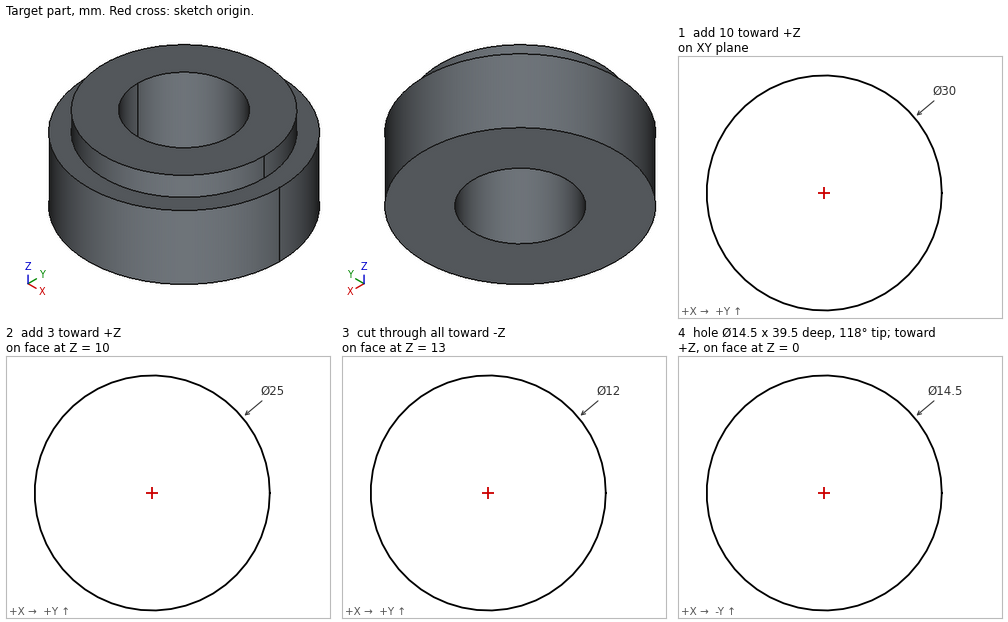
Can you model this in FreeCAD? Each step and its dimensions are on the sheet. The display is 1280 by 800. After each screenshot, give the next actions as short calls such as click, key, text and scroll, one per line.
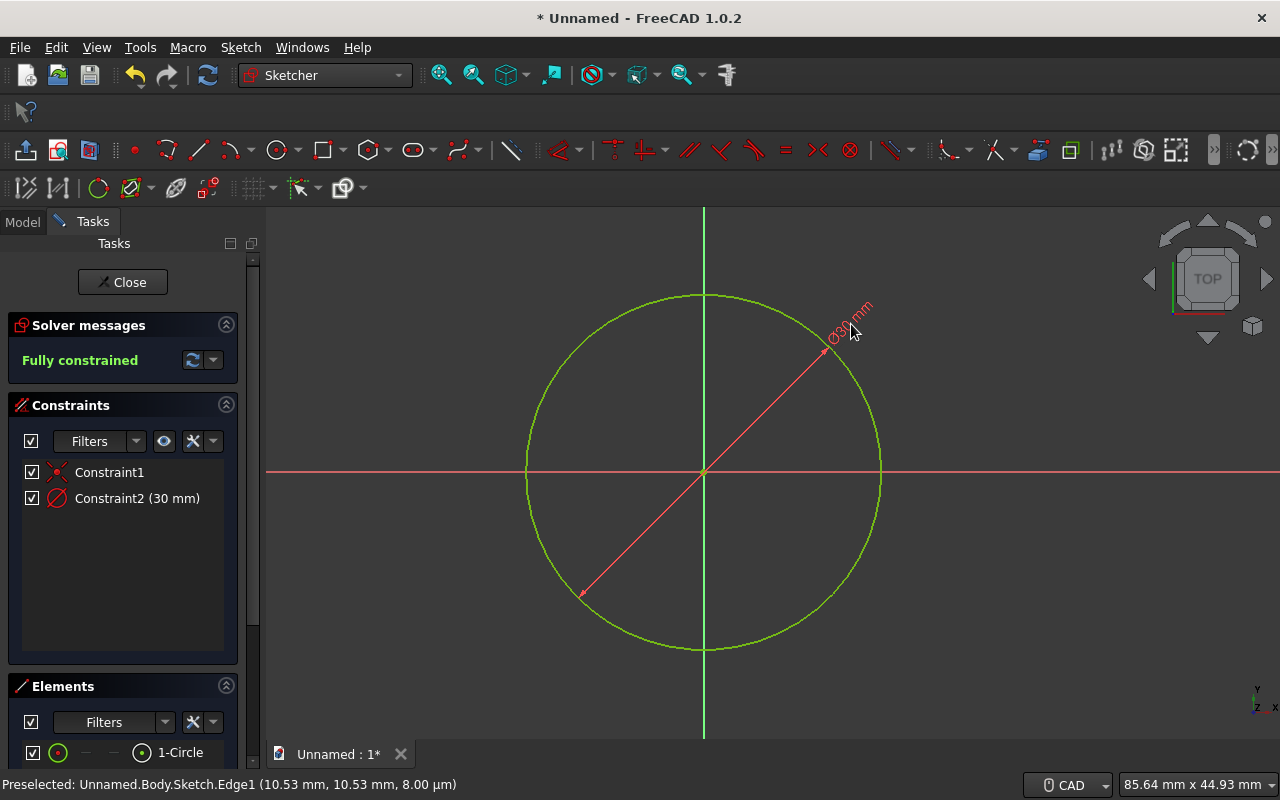
click(123, 282)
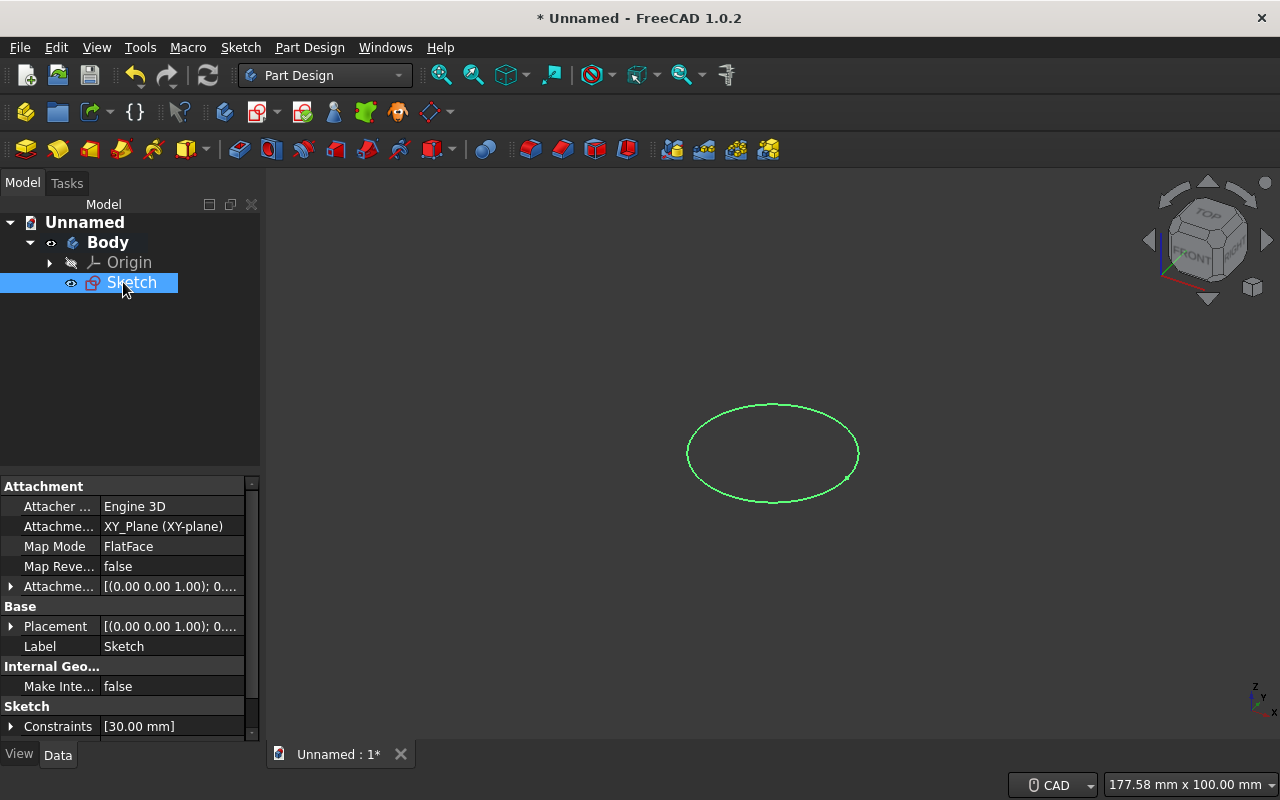
click(26, 150)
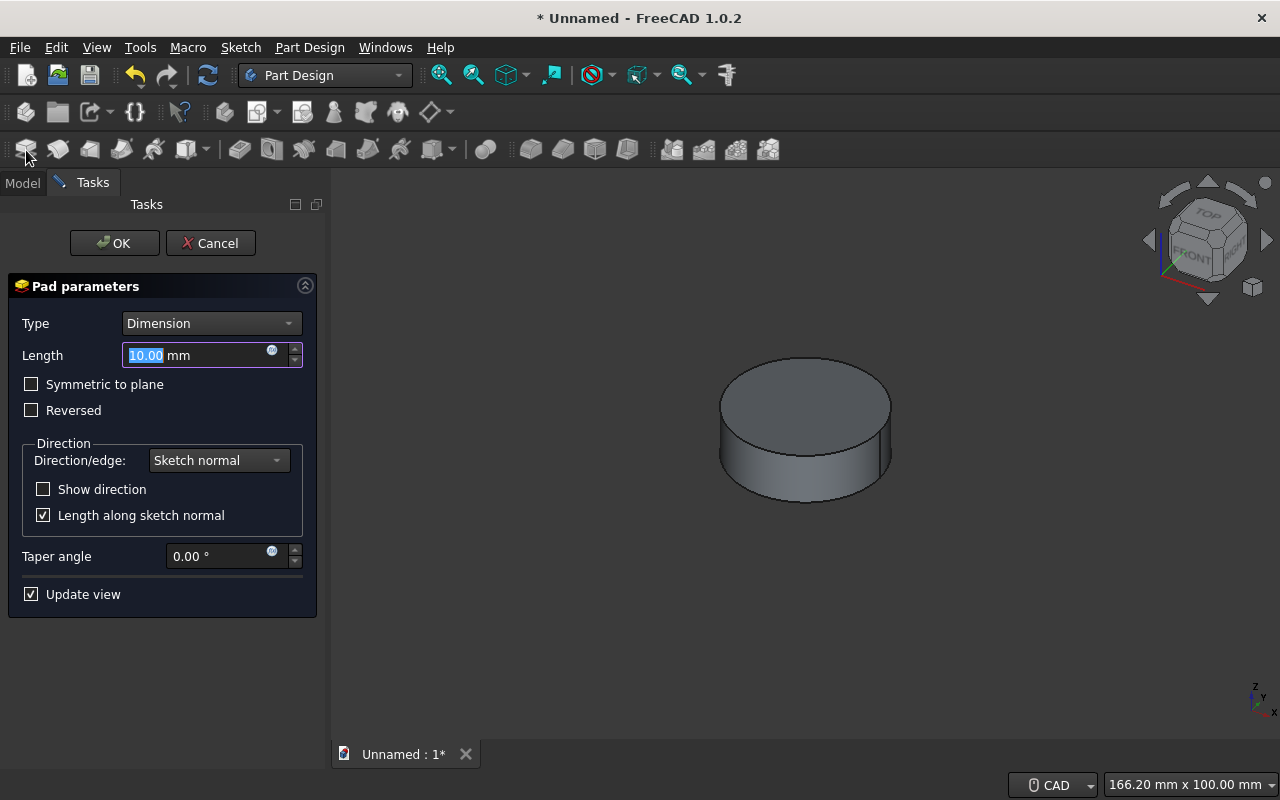
text(10)
key(Tab)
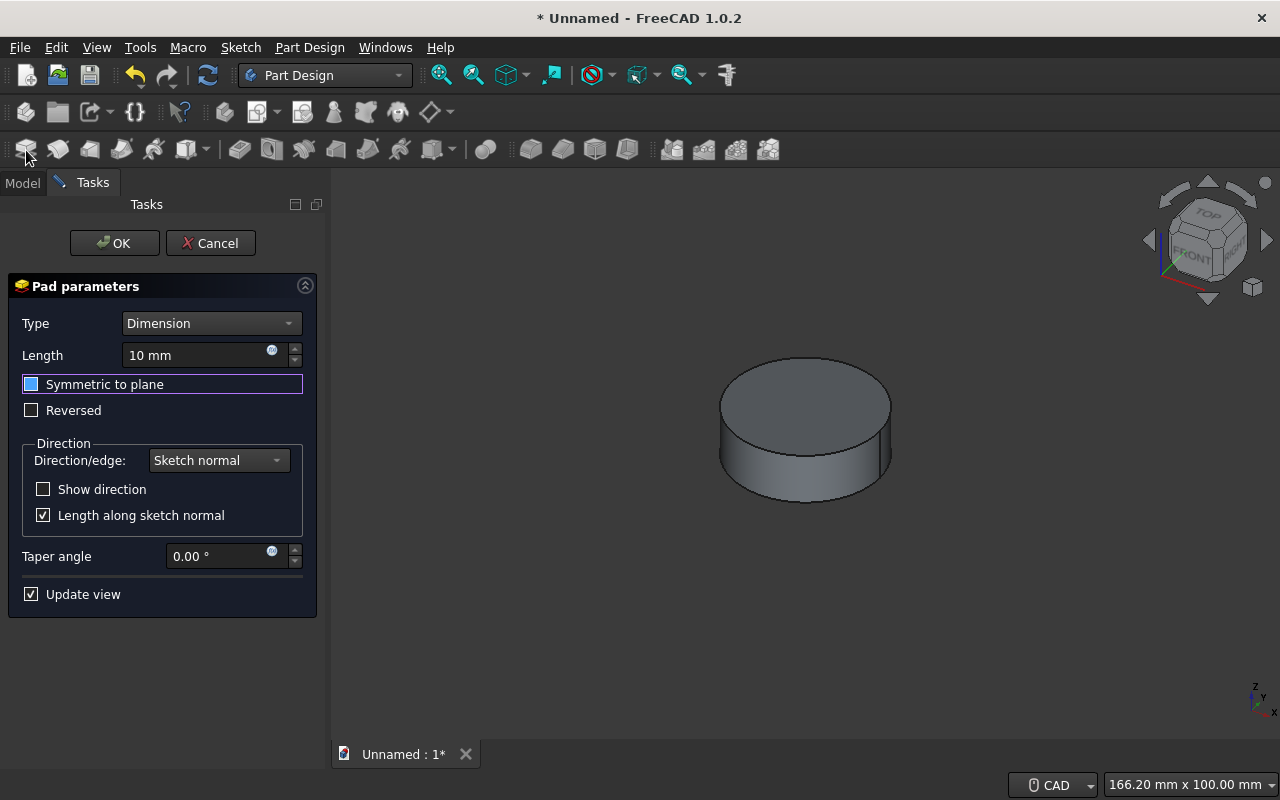
click(115, 243)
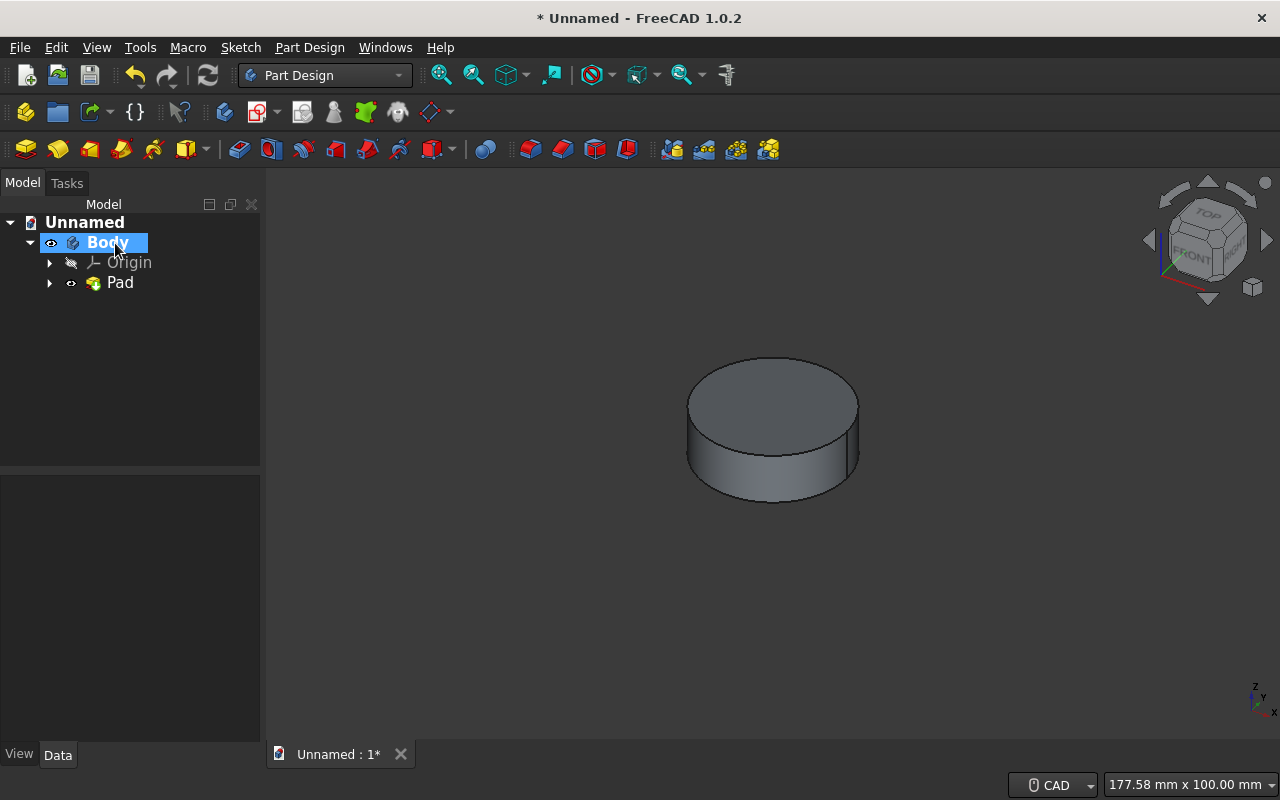
click(442, 76)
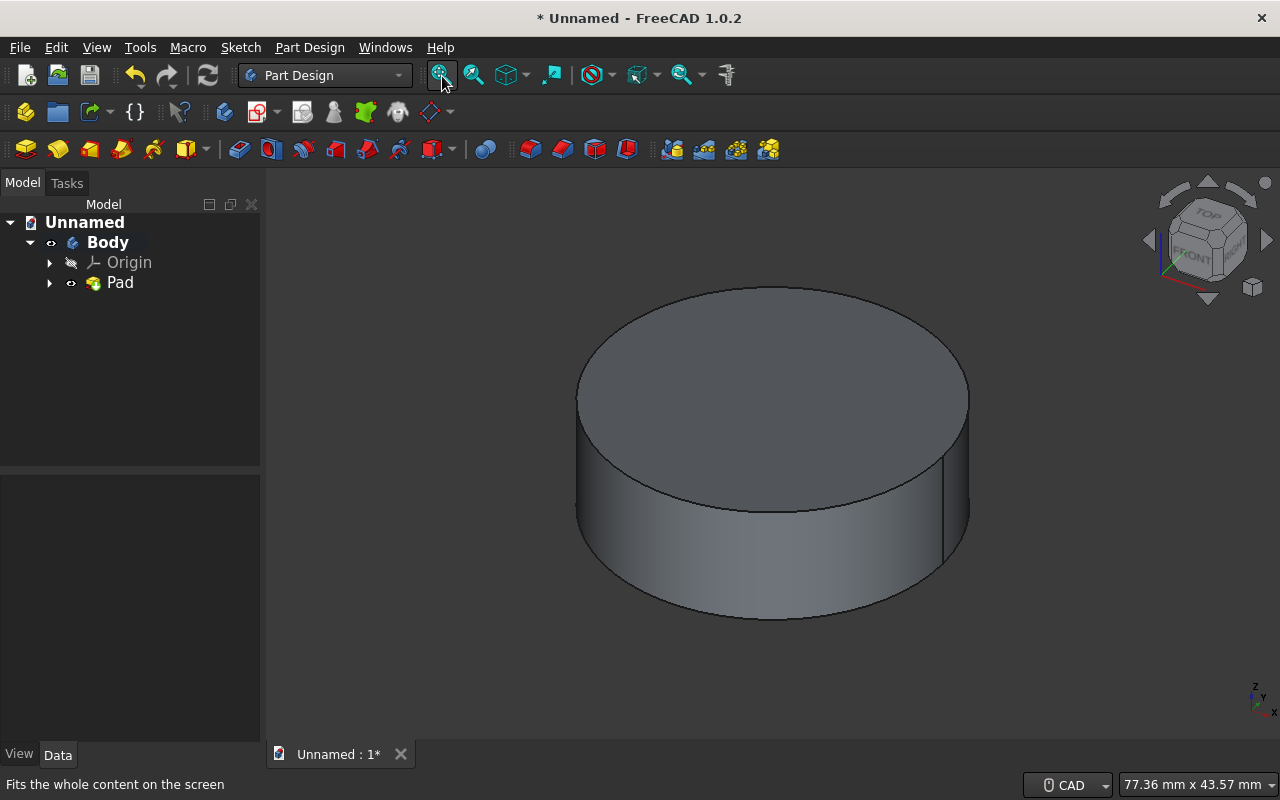
click(773, 399)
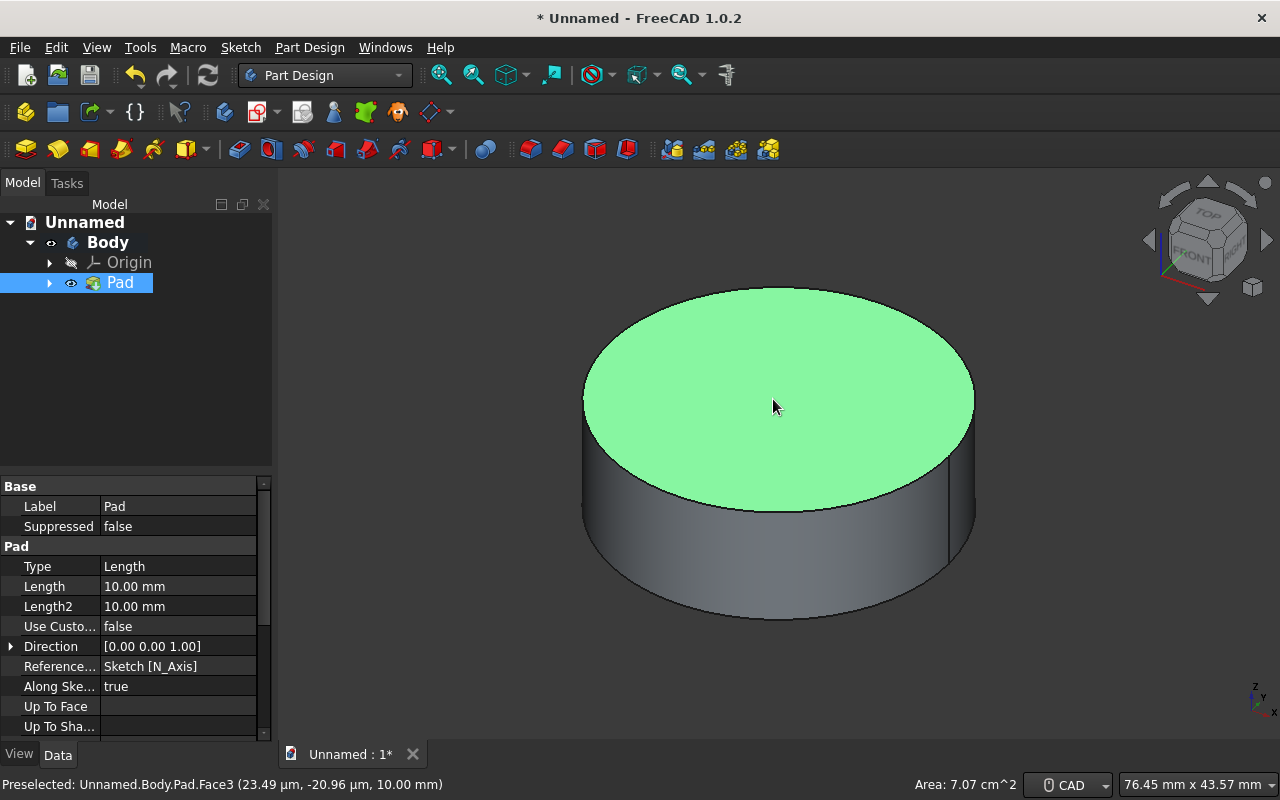
click(258, 112)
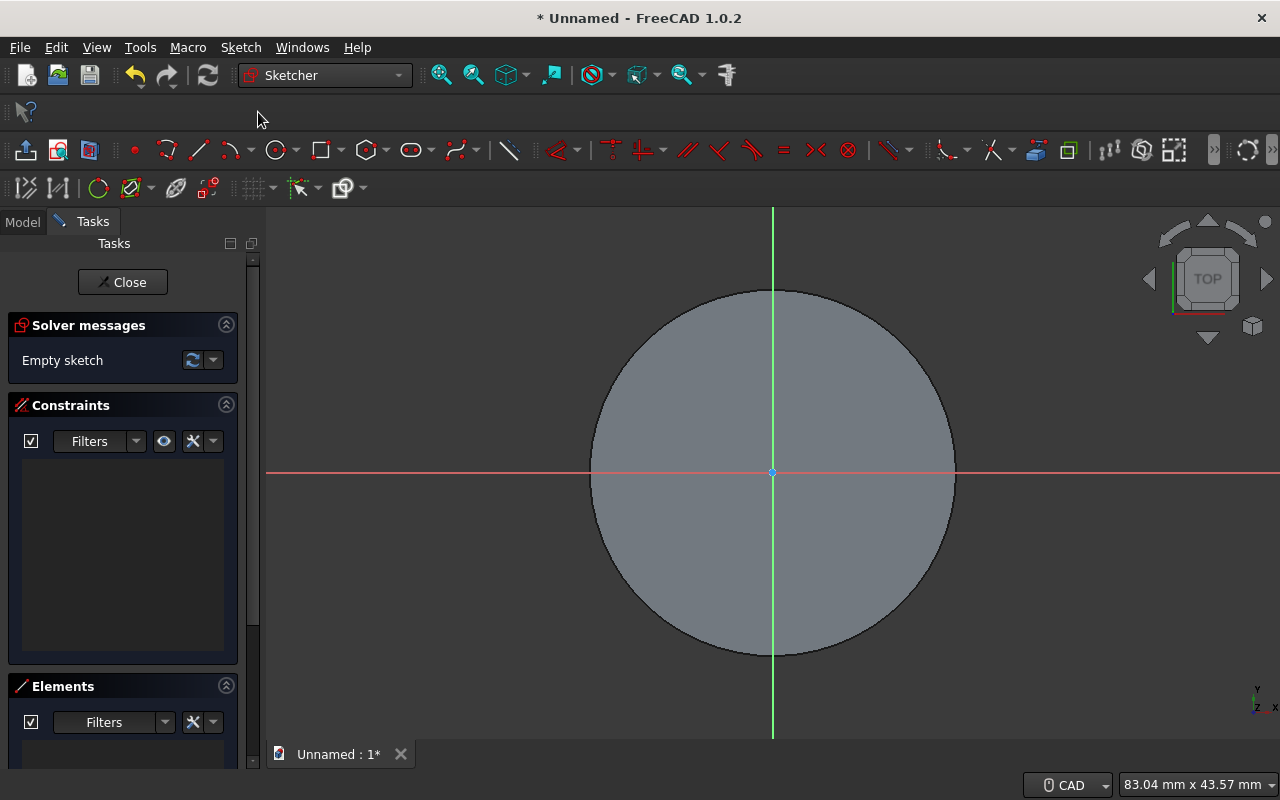
click(276, 150)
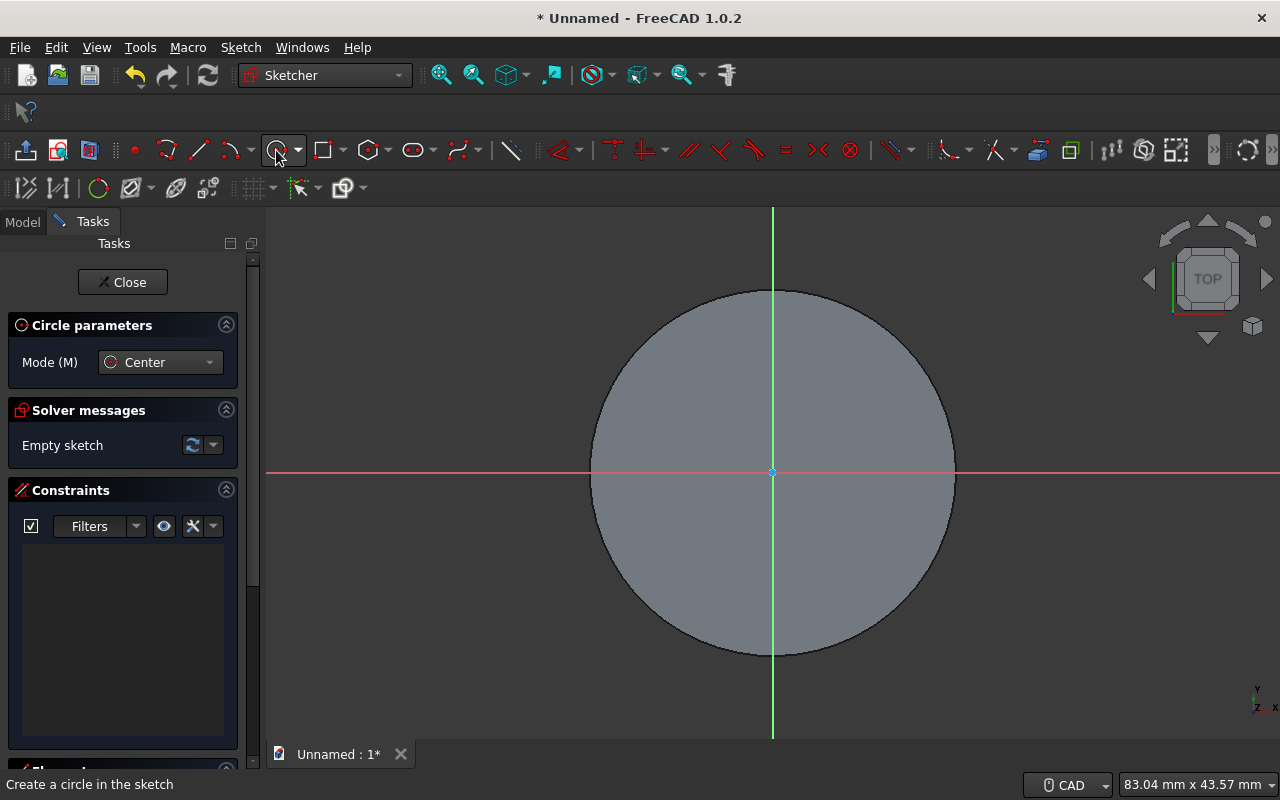
click(773, 473)
click(881, 365)
key(Escape)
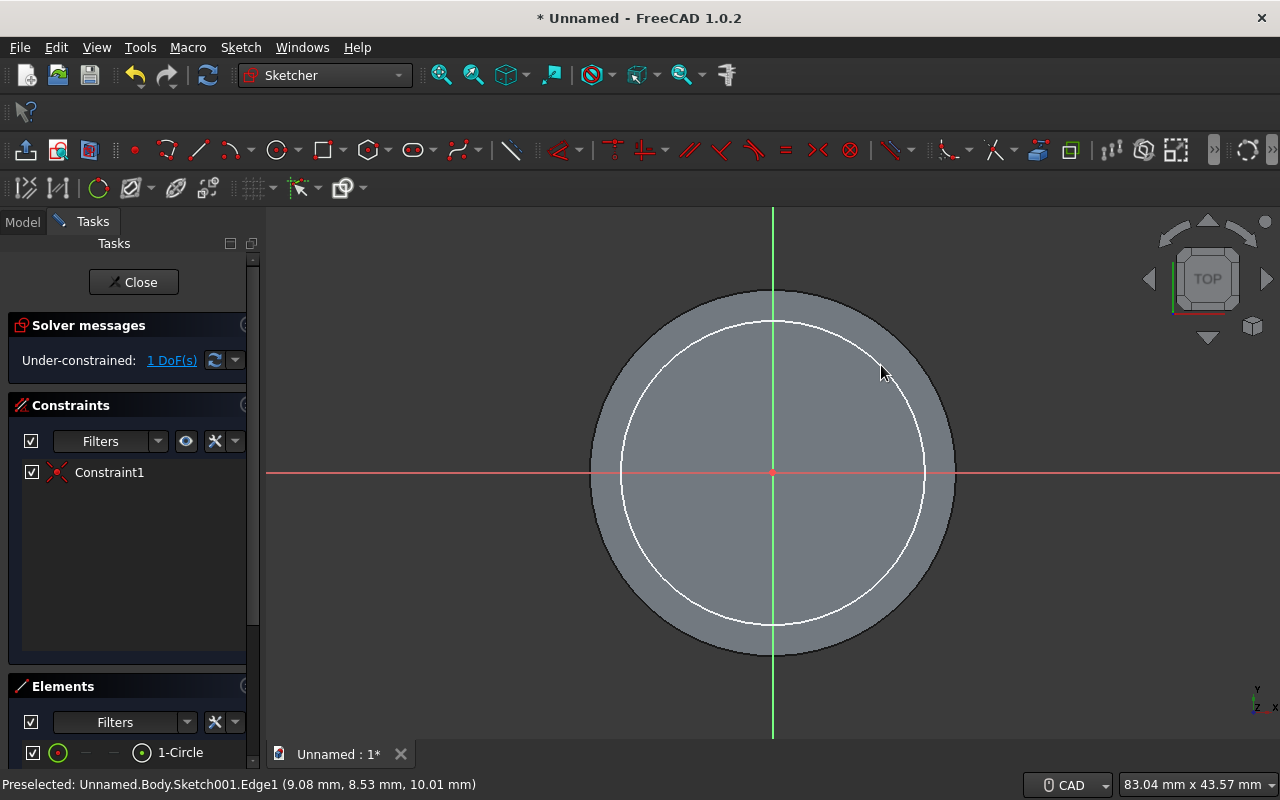
click(558, 150)